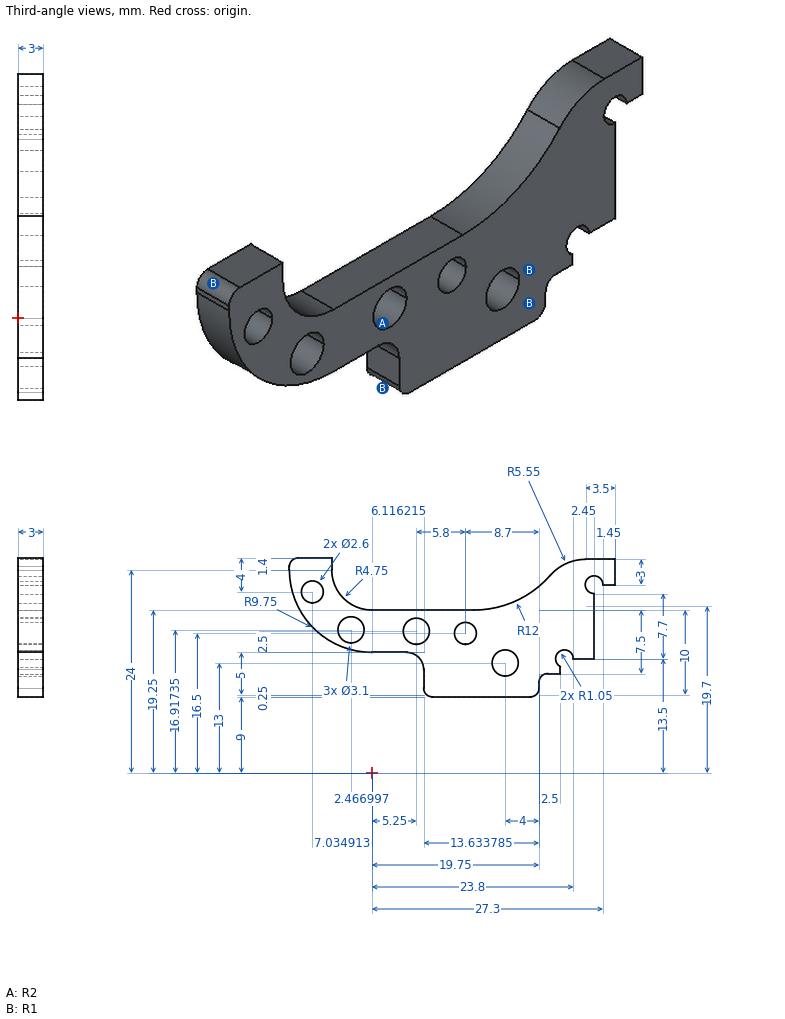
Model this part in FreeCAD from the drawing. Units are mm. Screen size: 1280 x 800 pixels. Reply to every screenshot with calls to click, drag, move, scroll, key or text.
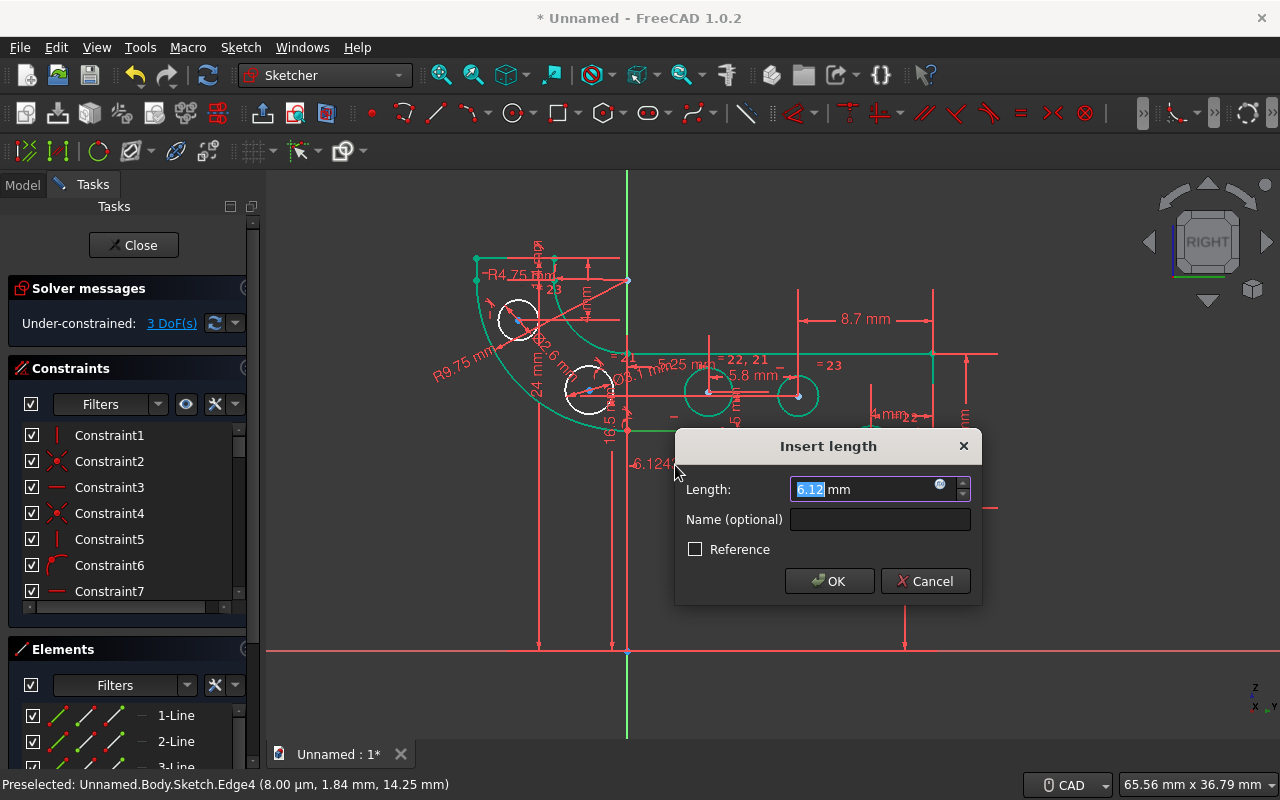
text(6.116215)
key(Return)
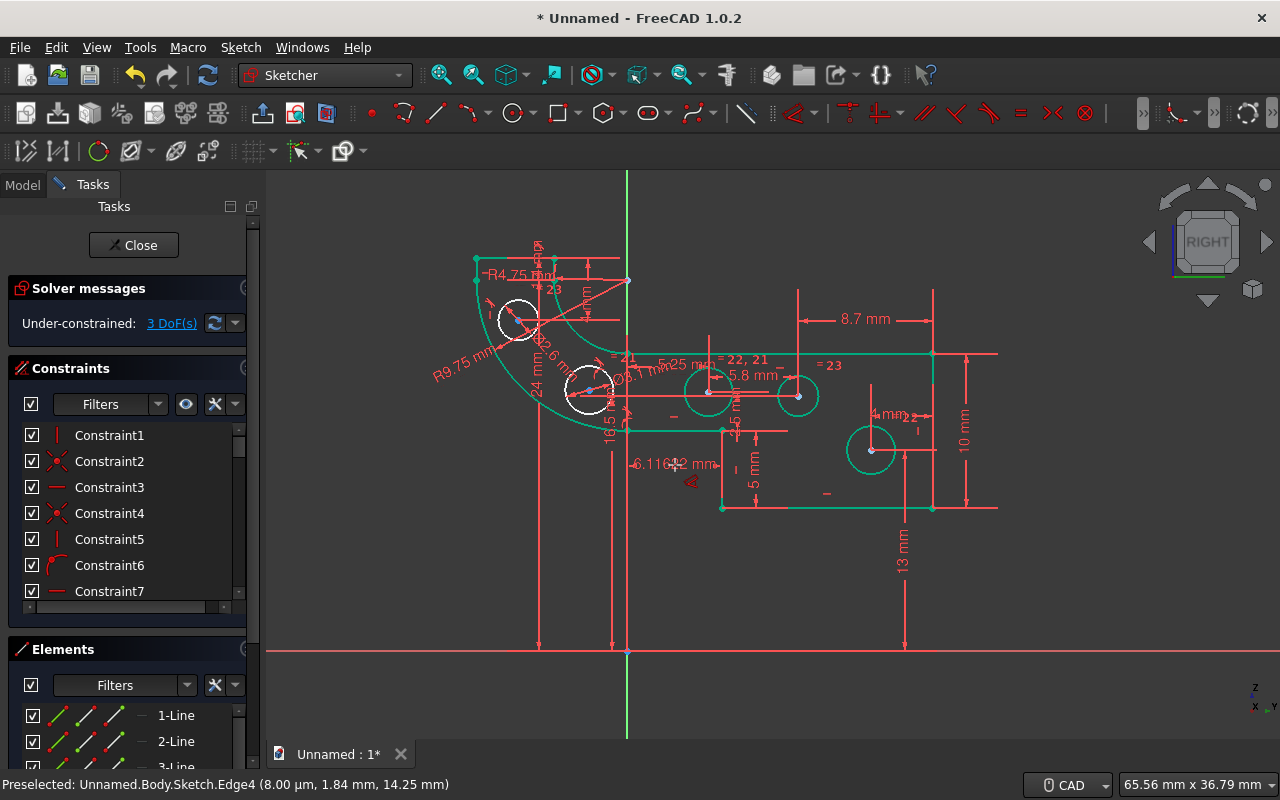
click(519, 320)
click(573, 685)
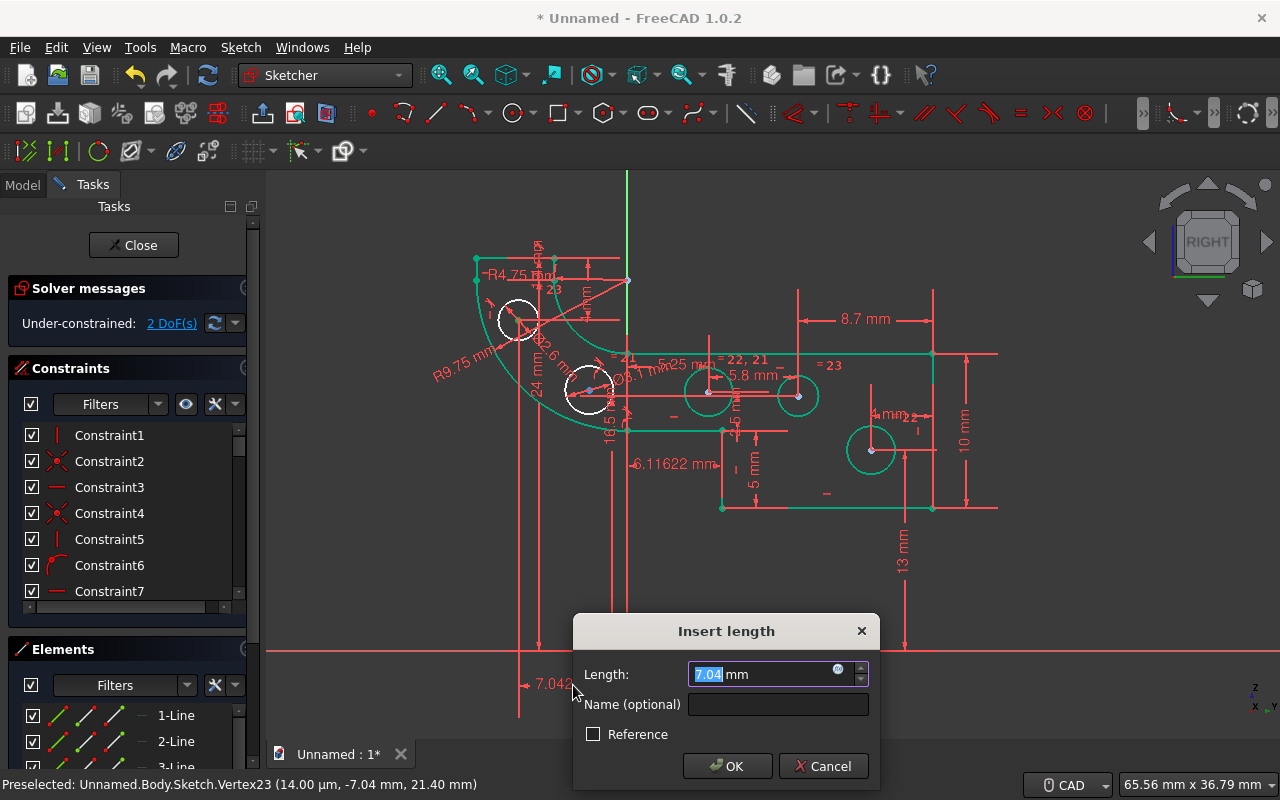
text(7.034913)
key(Return)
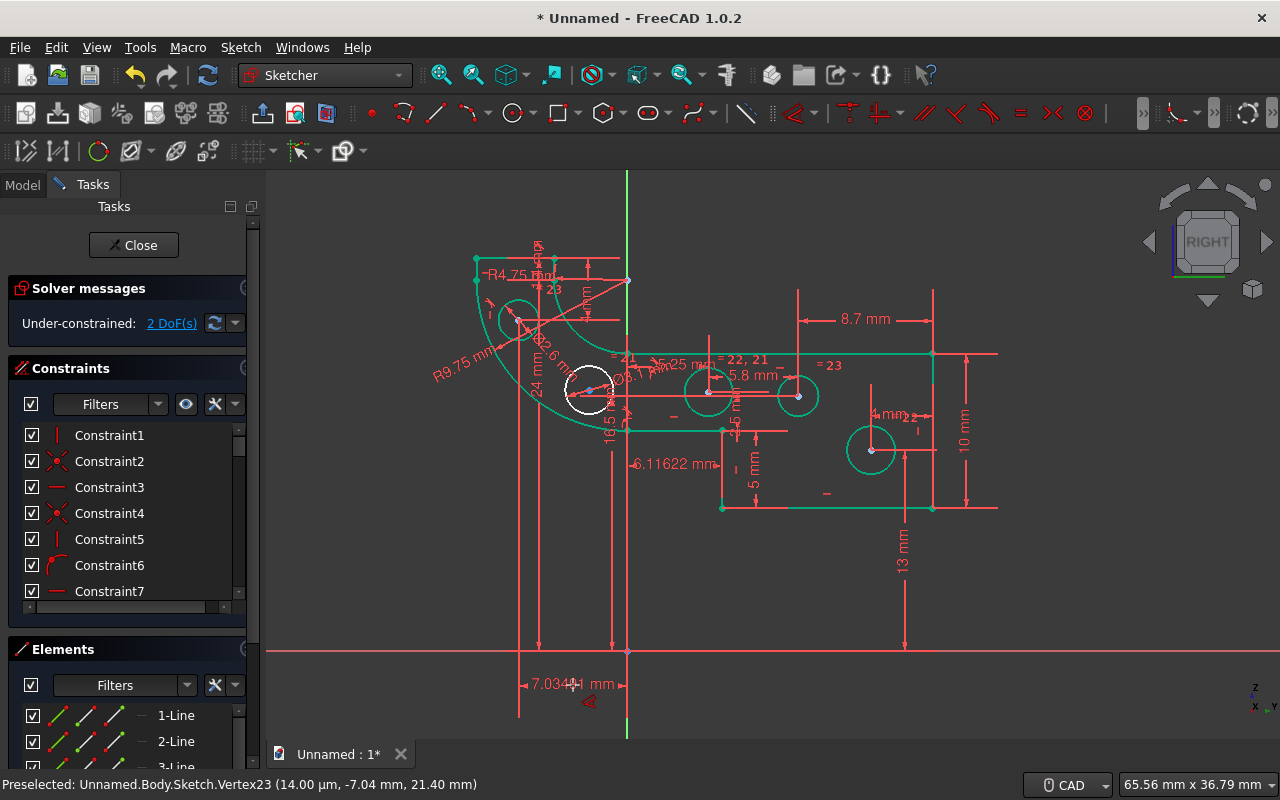
click(589, 390)
click(608, 709)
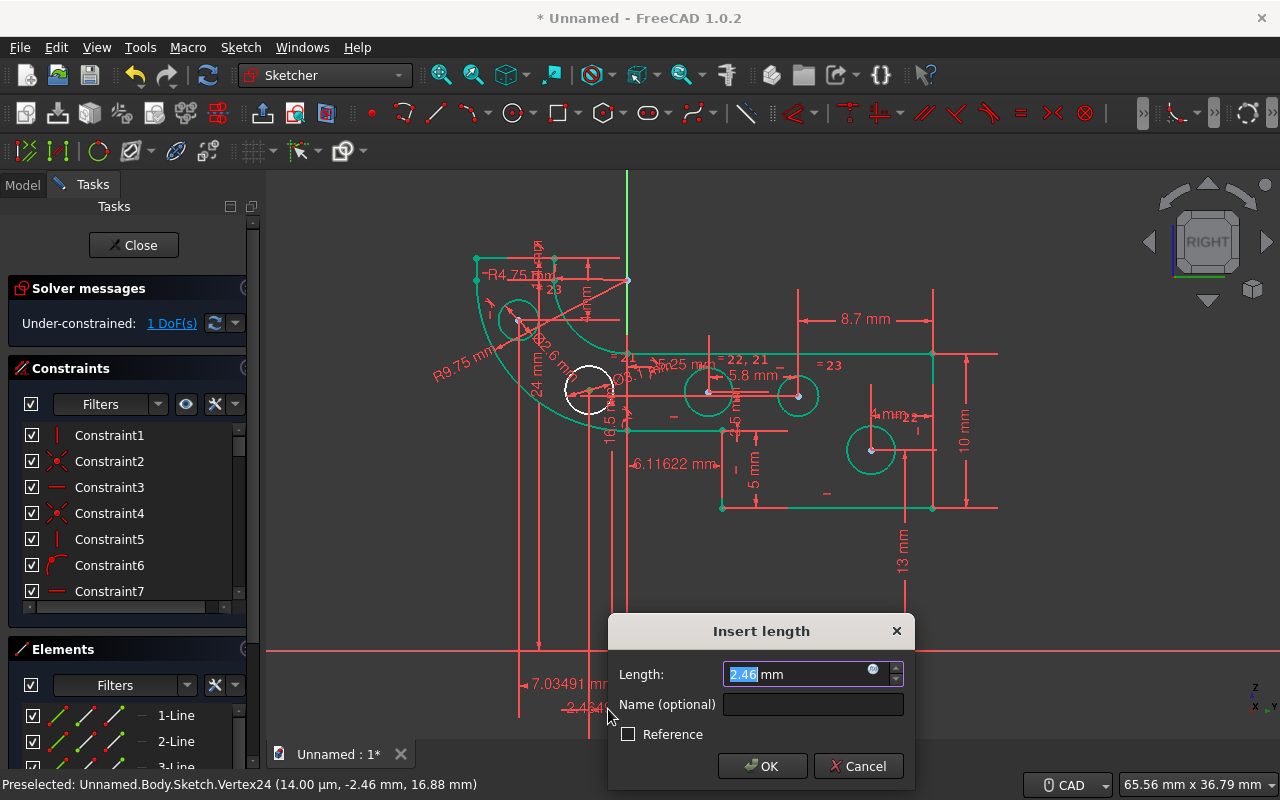
text(2.466997)
key(Return)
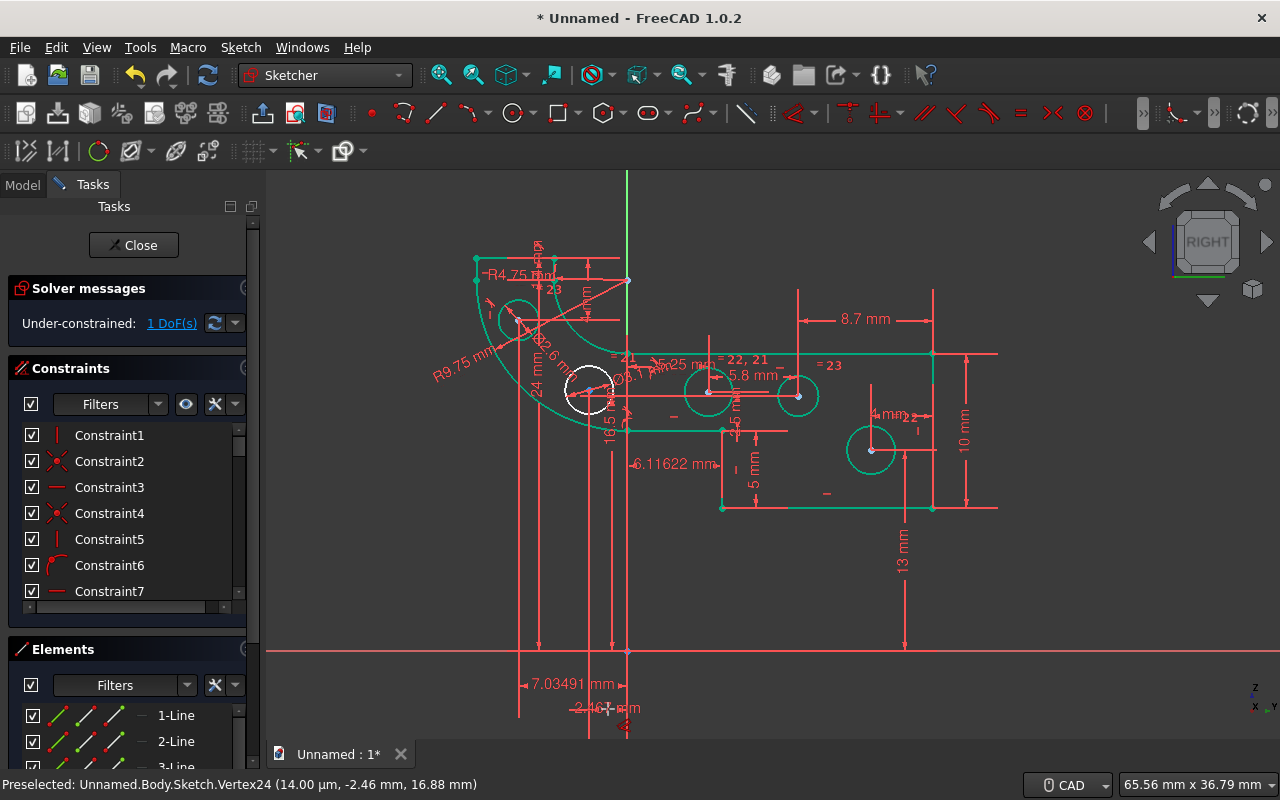
click(589, 390)
click(555, 521)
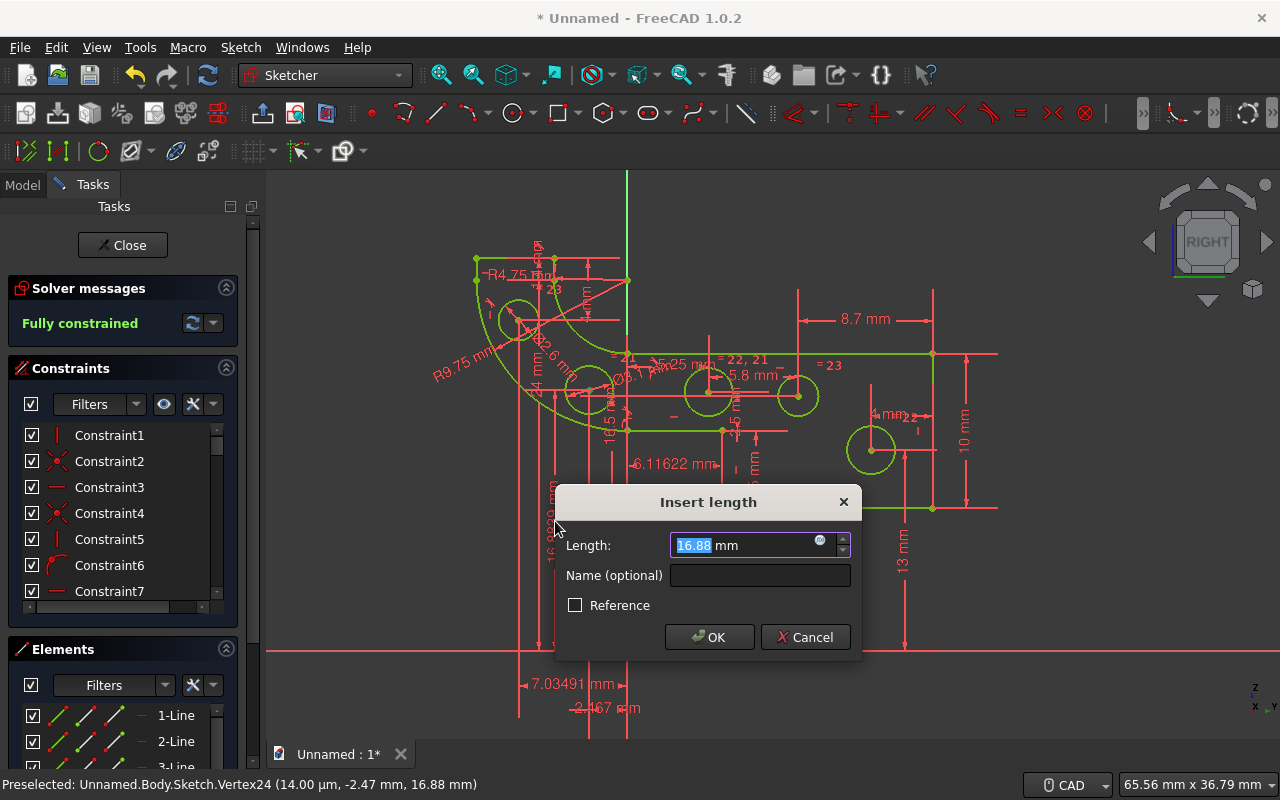
text(16.91735)
key(Return)
key(Escape)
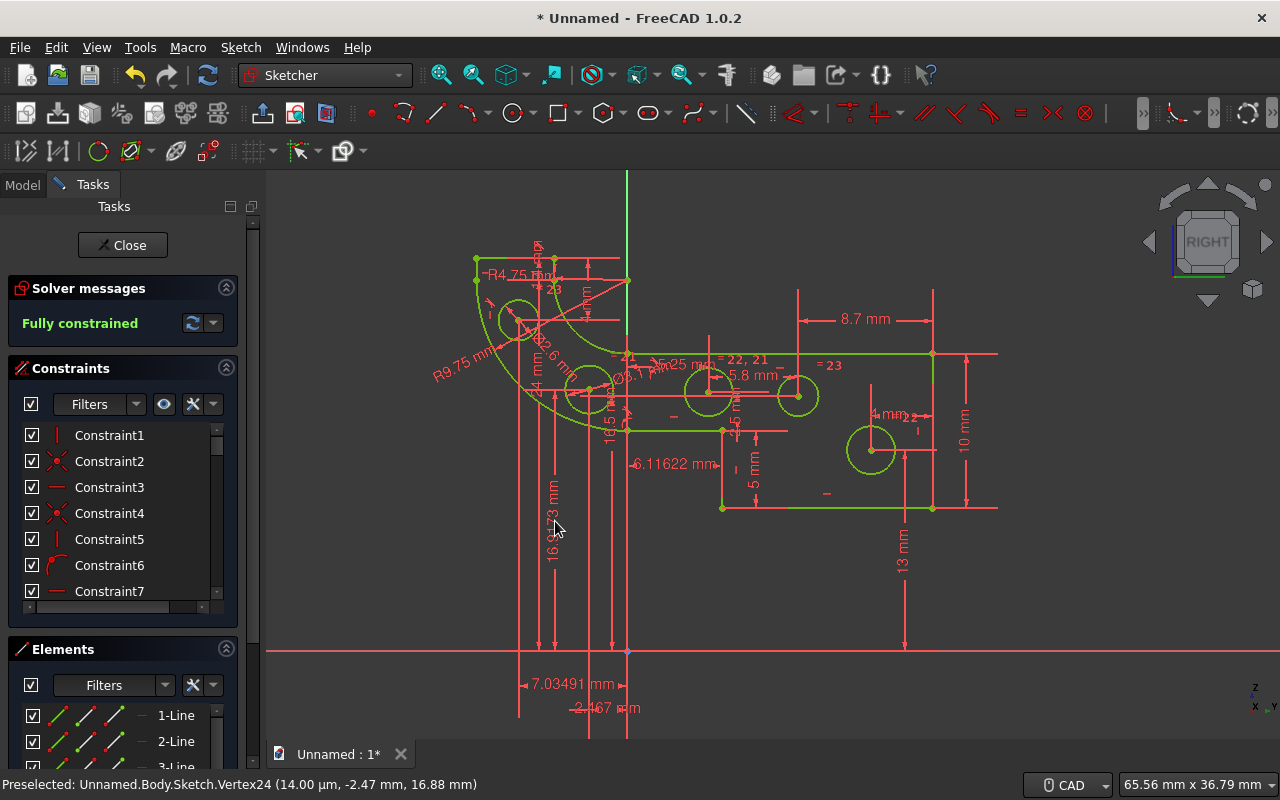
click(123, 245)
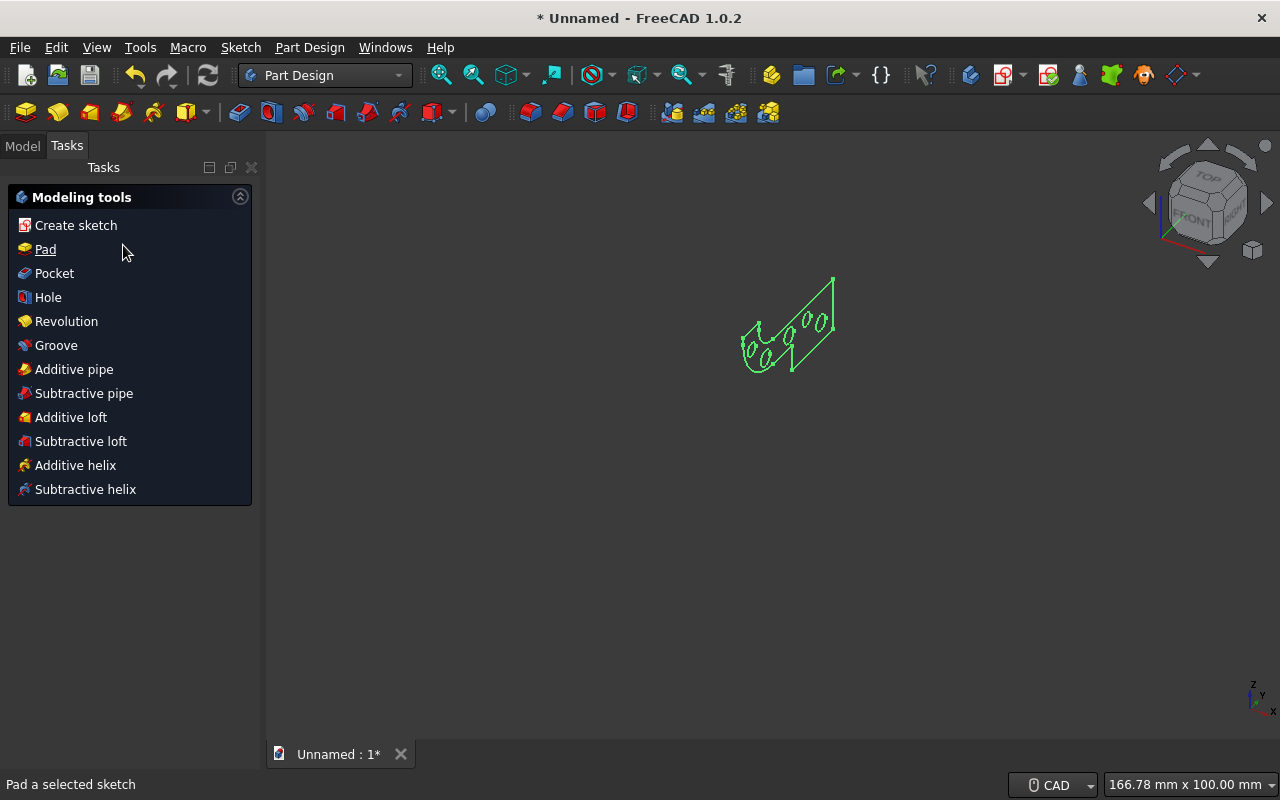
click(26, 112)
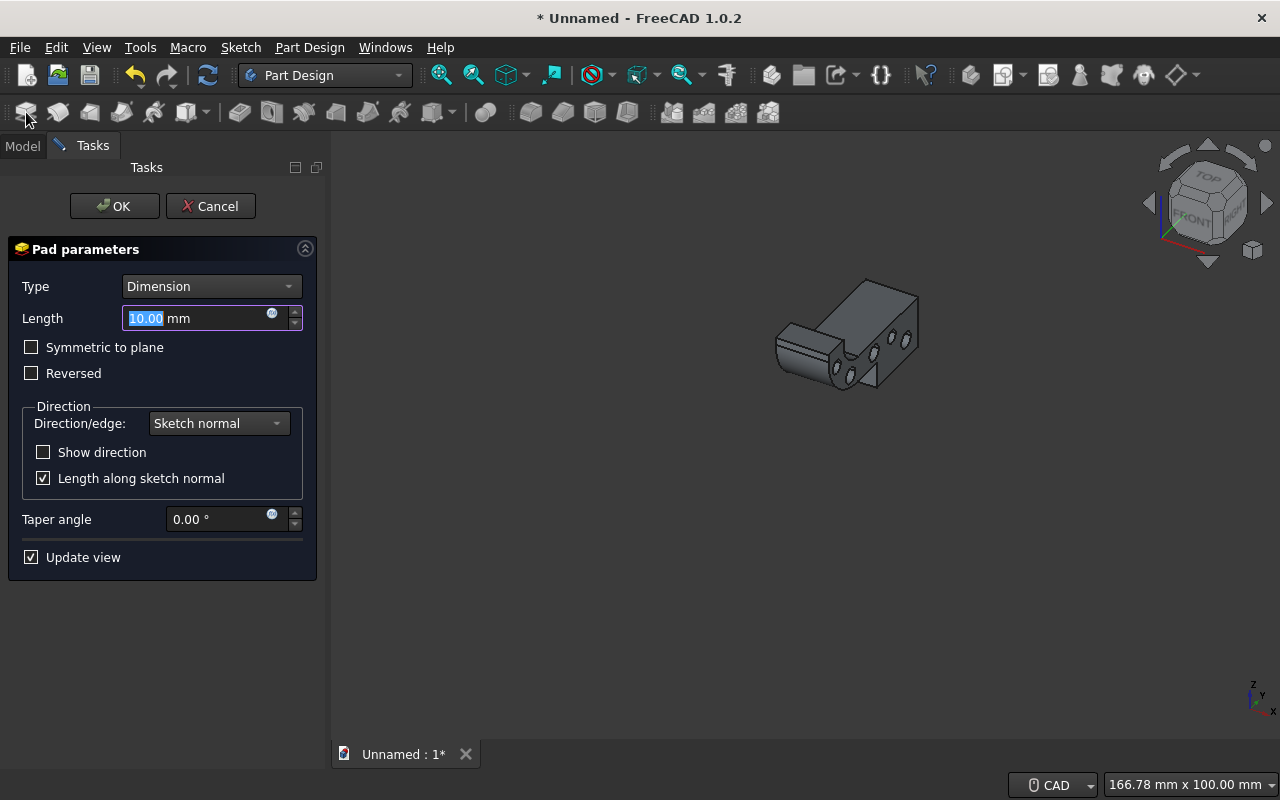
text(3)
key(Tab)